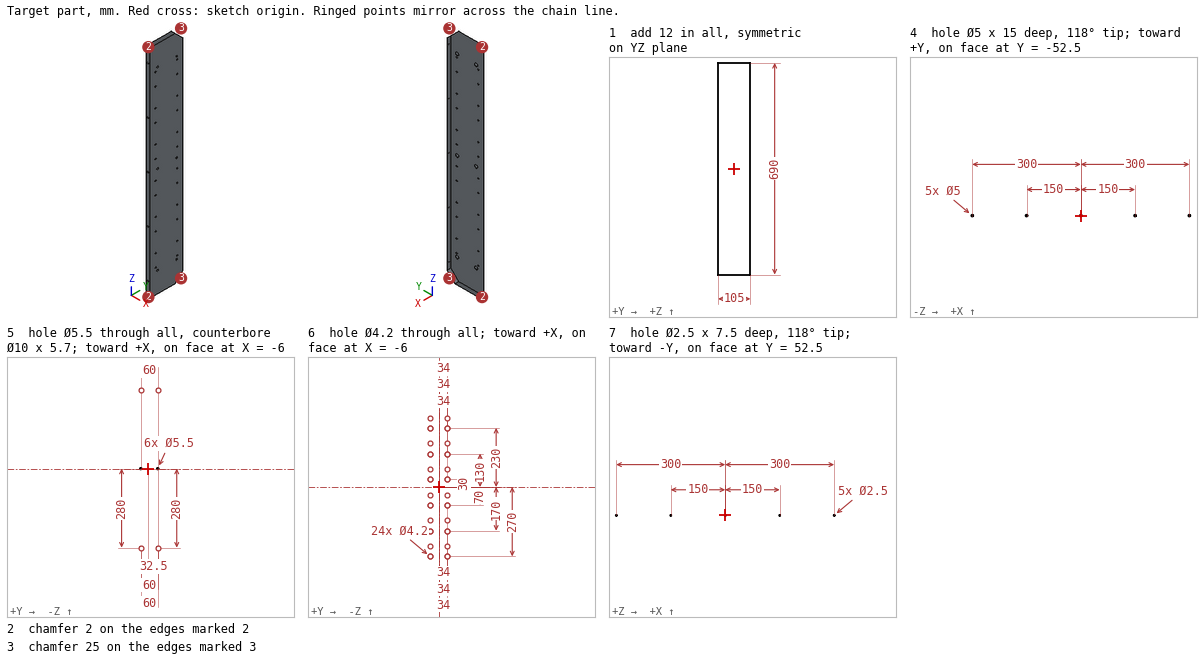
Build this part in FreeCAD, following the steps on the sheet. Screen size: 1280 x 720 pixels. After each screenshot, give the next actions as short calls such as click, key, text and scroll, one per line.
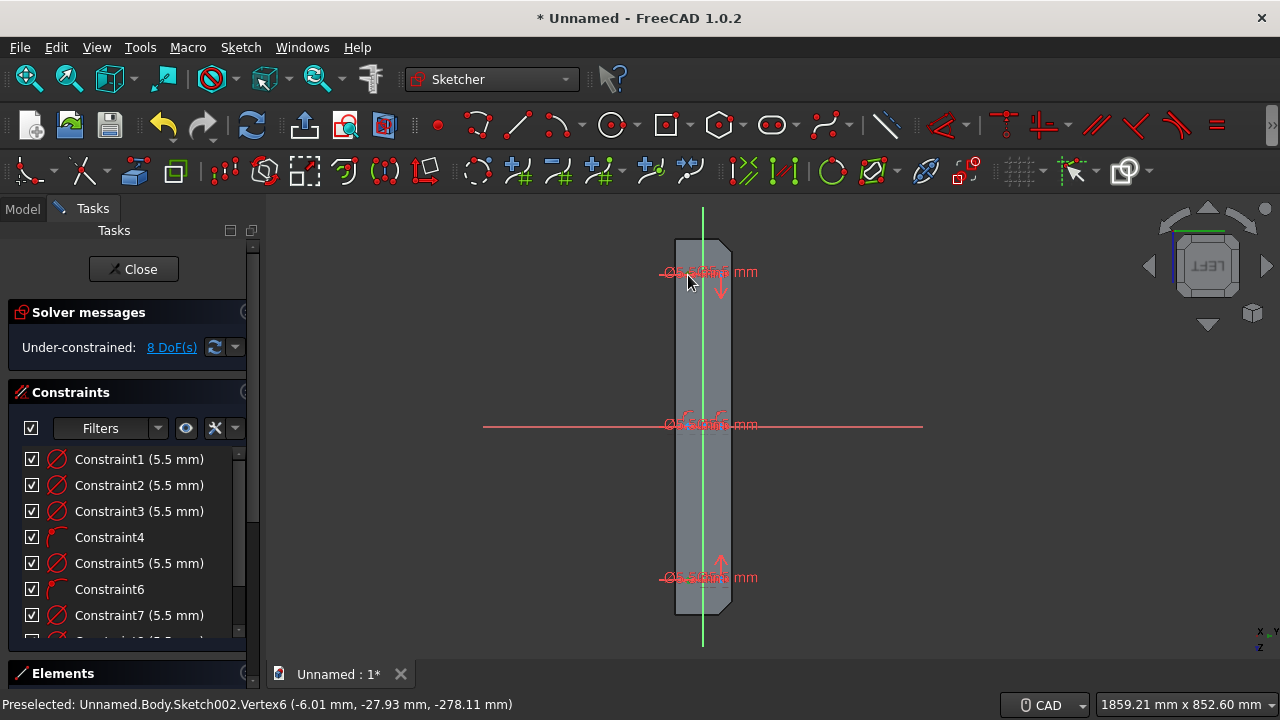
click(529, 427)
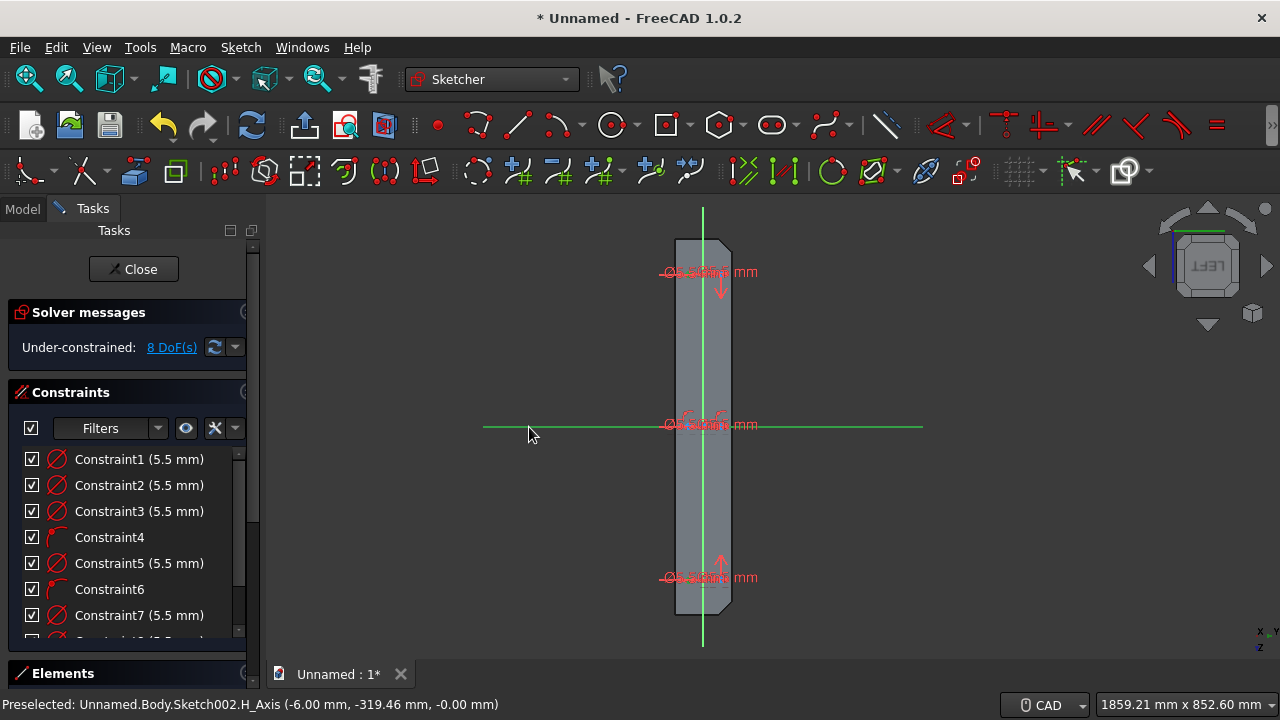
key(s)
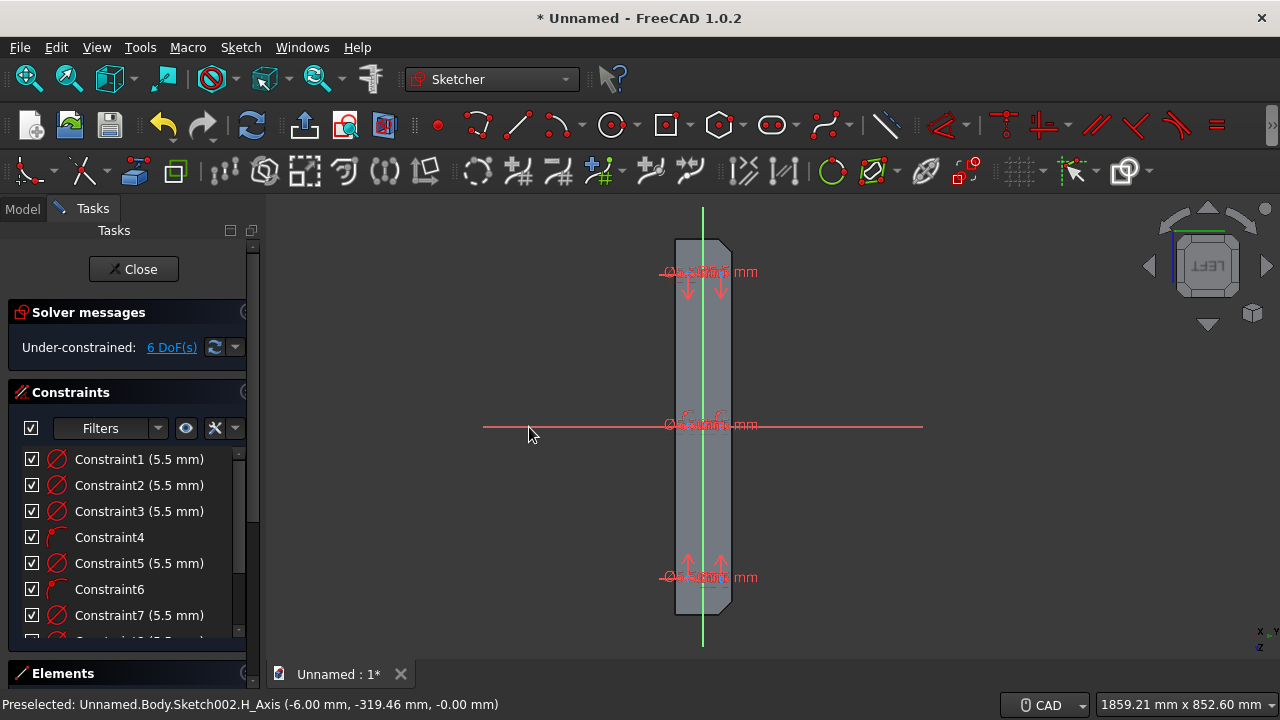
click(942, 126)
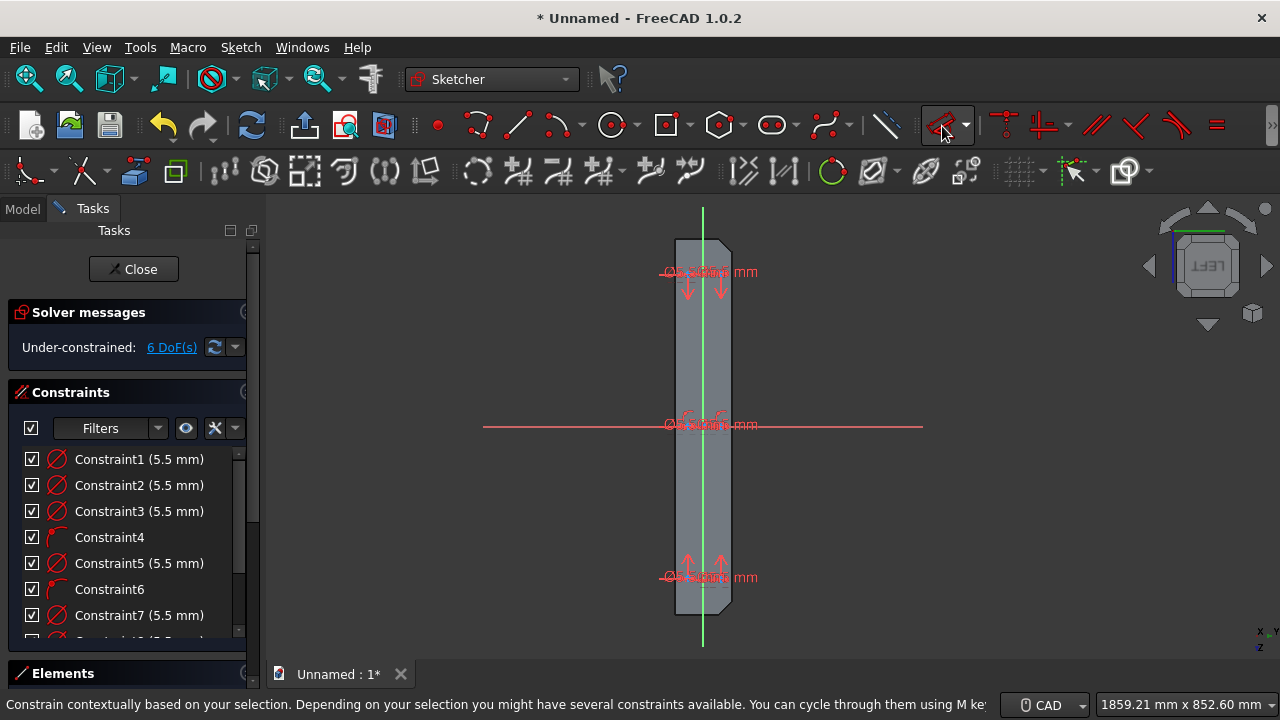
click(721, 580)
click(755, 503)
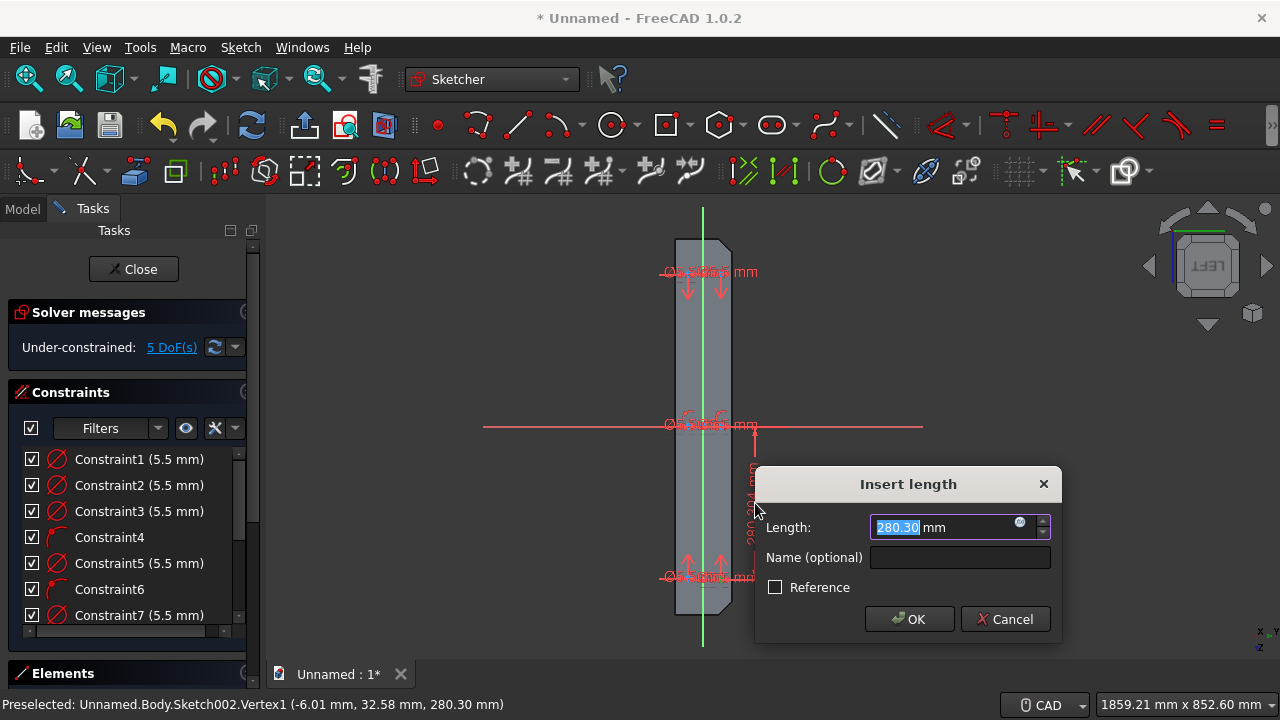
text(280)
key(Return)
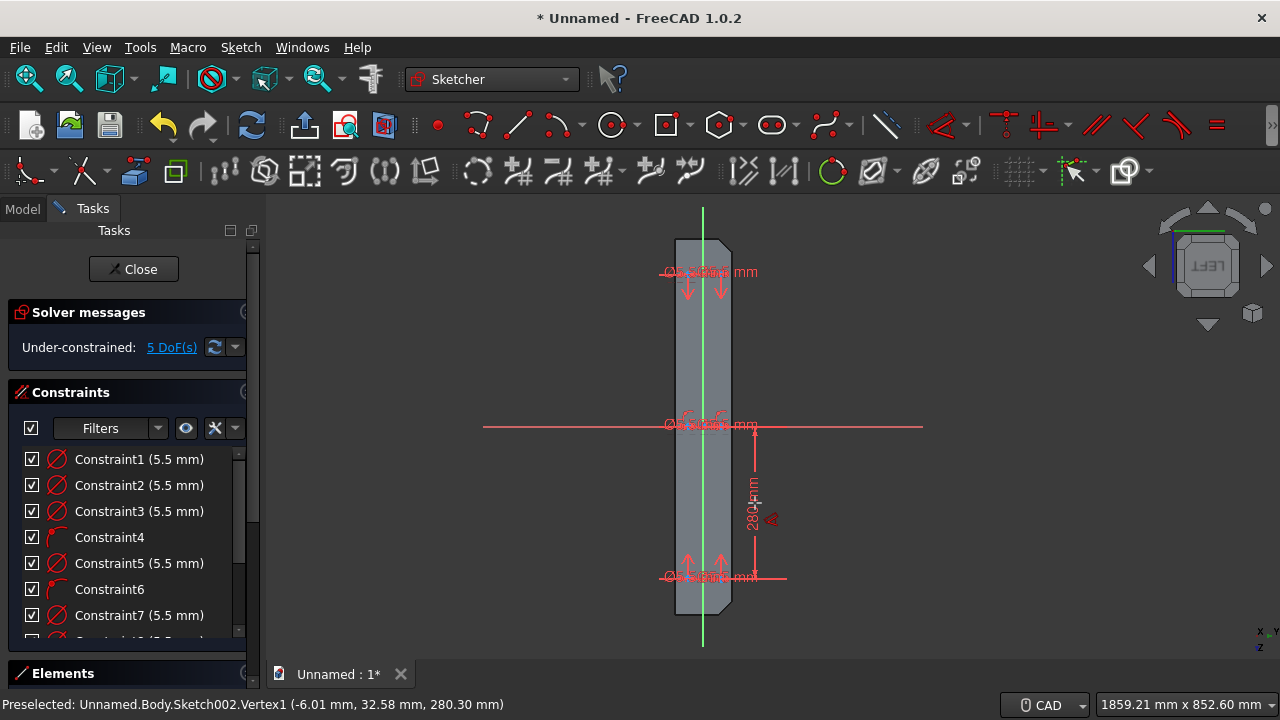
click(688, 579)
click(654, 503)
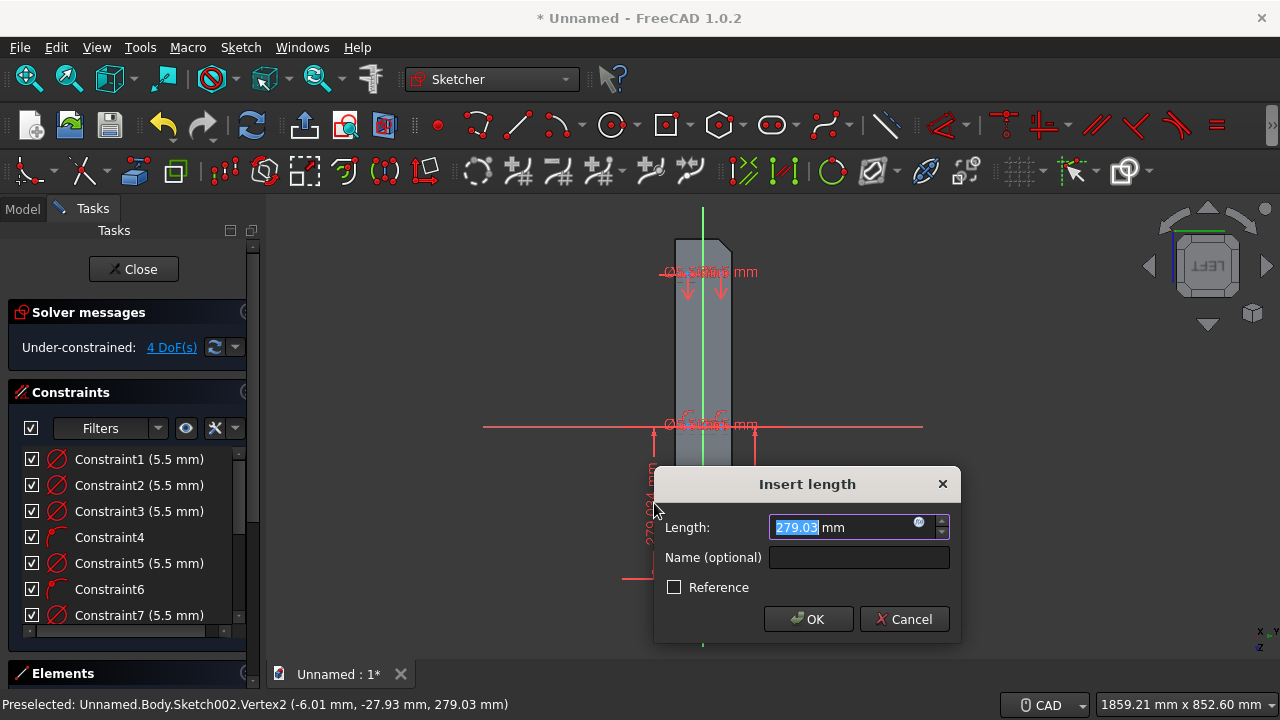
text(280)
key(Return)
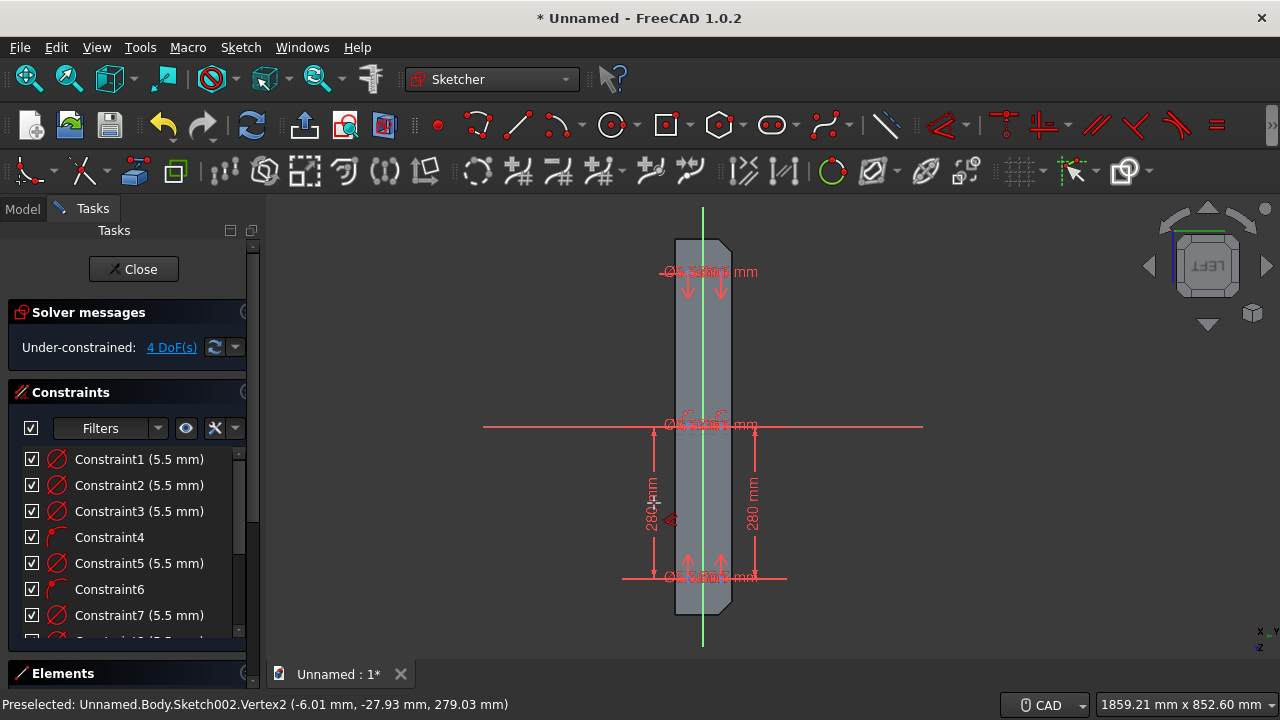
click(721, 579)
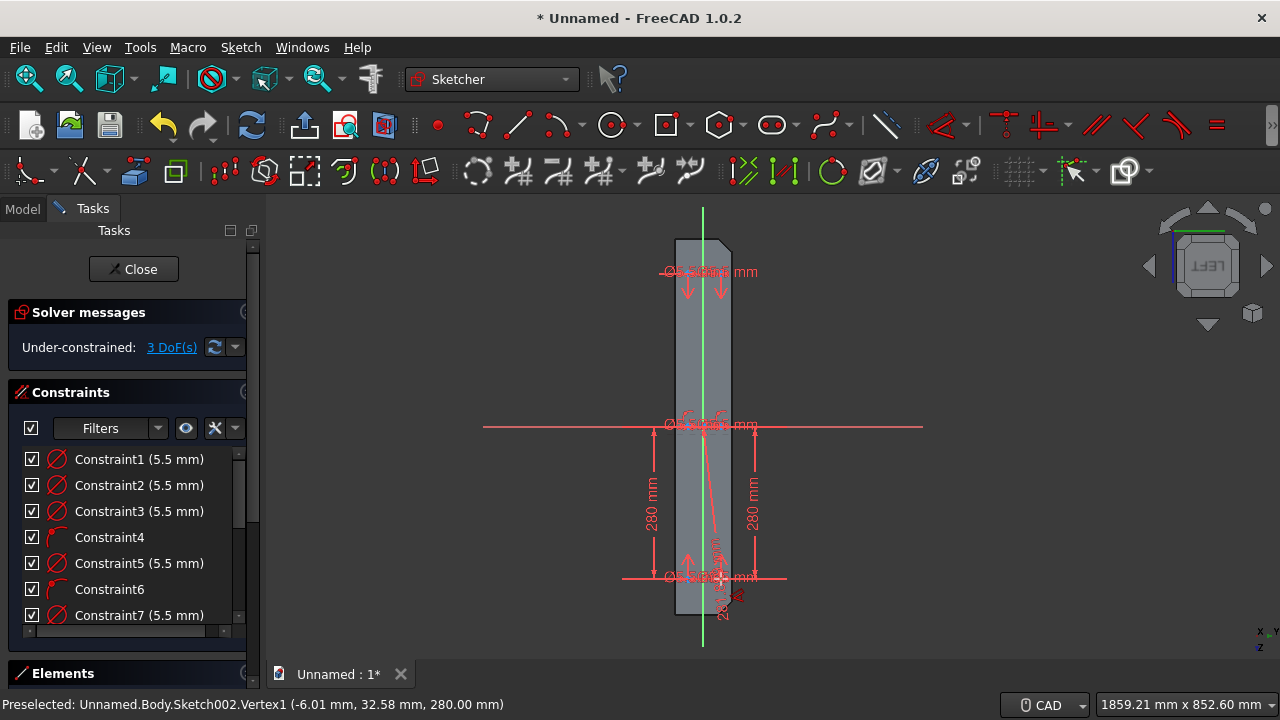
click(688, 579)
click(712, 613)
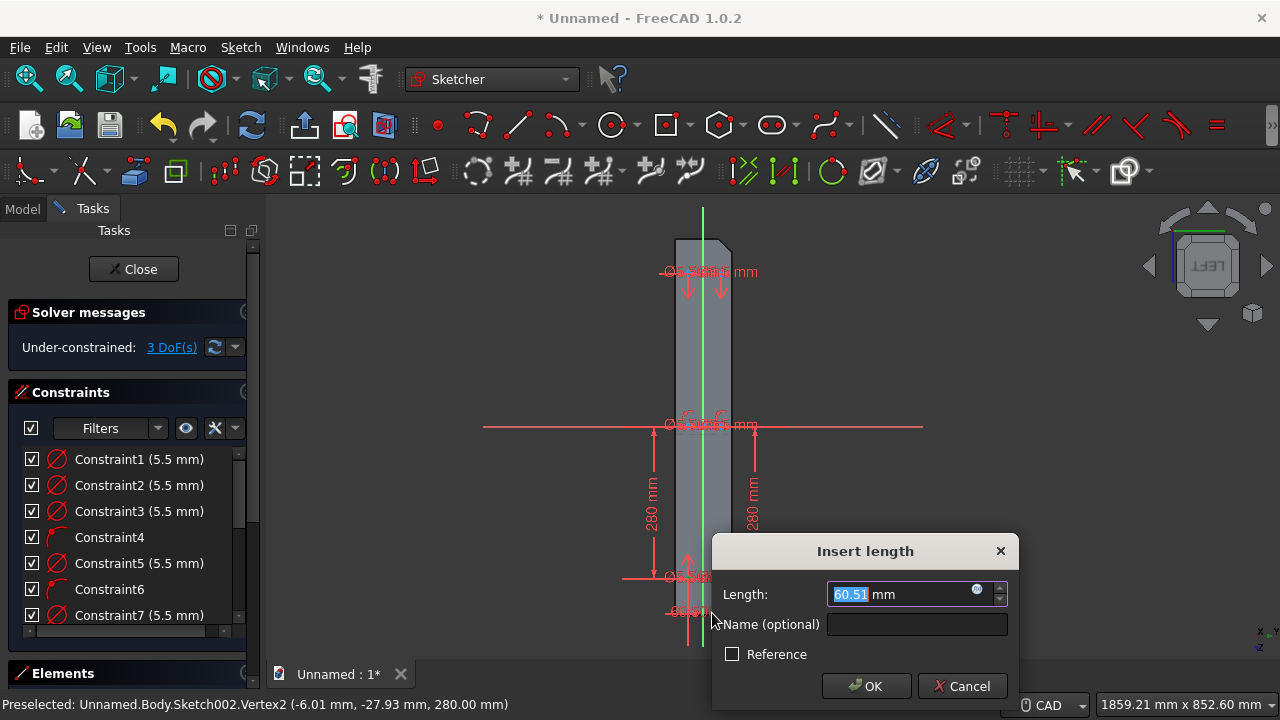
text(60)
key(Return)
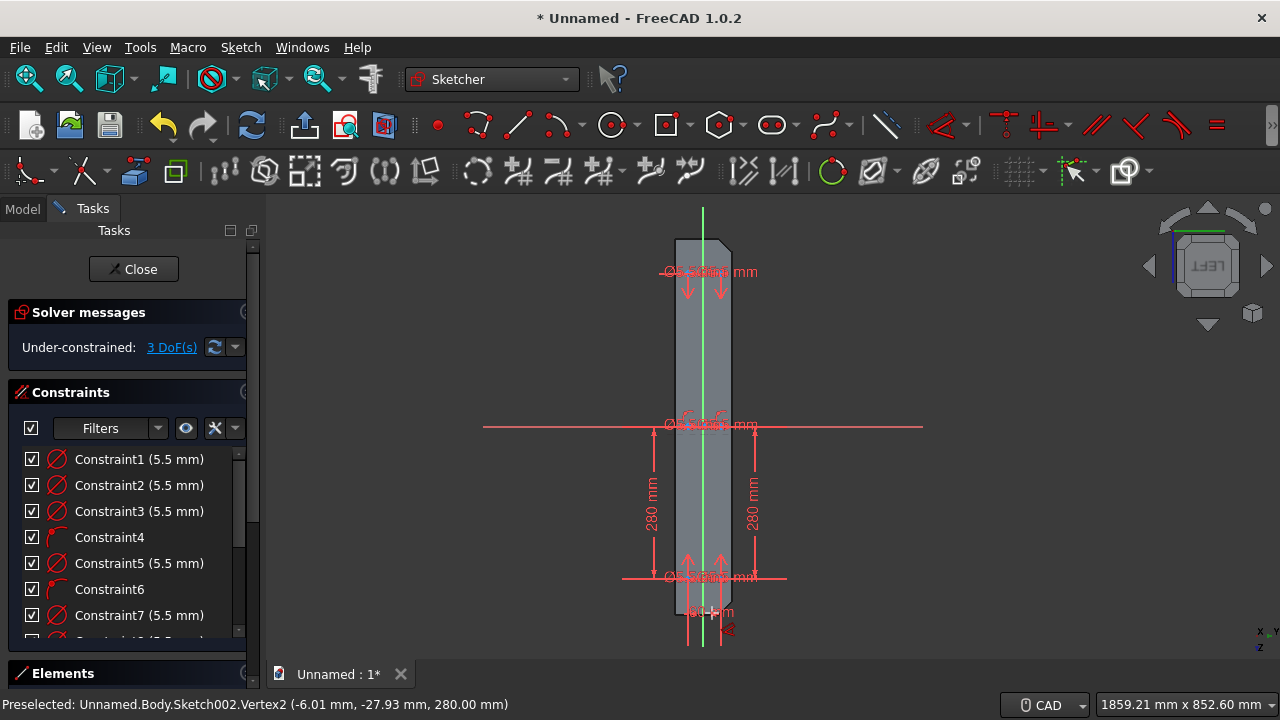
click(688, 579)